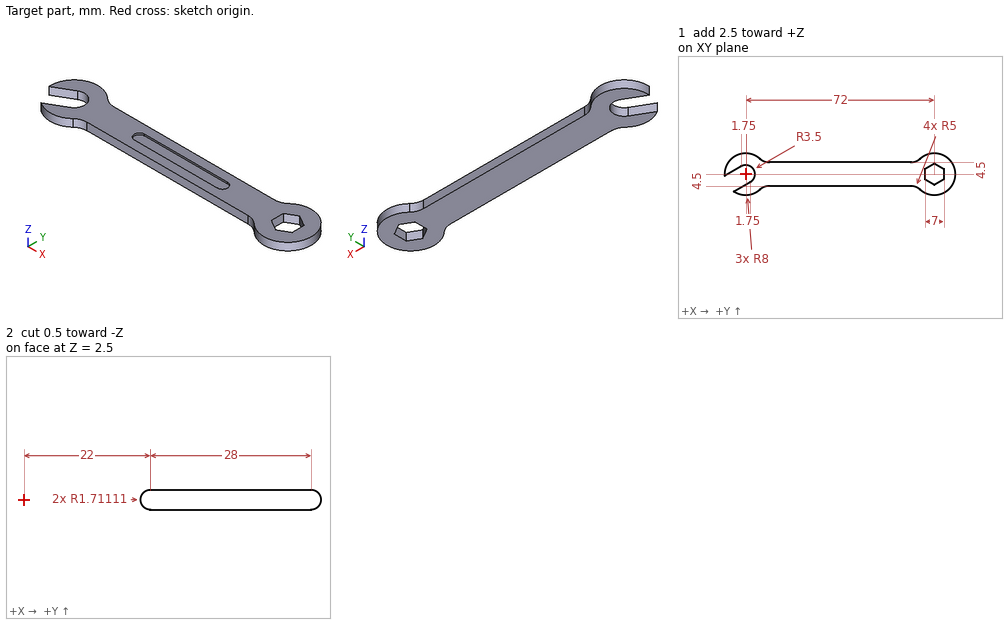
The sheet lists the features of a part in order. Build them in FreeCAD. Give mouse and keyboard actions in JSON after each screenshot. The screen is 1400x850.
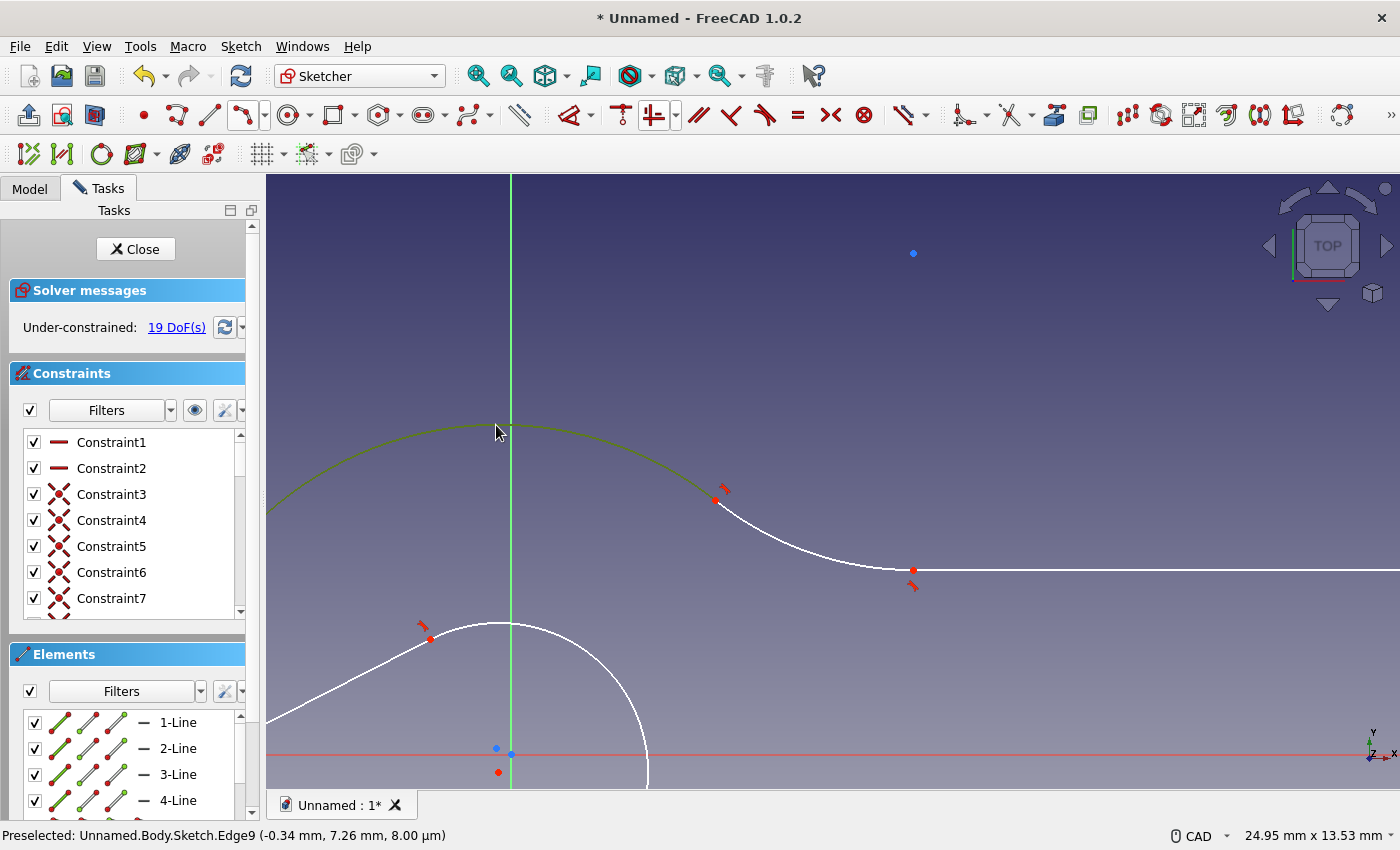
{"action": "scroll", "coordinate": [491, 424], "scroll_direction": "down", "scroll_amount": 9}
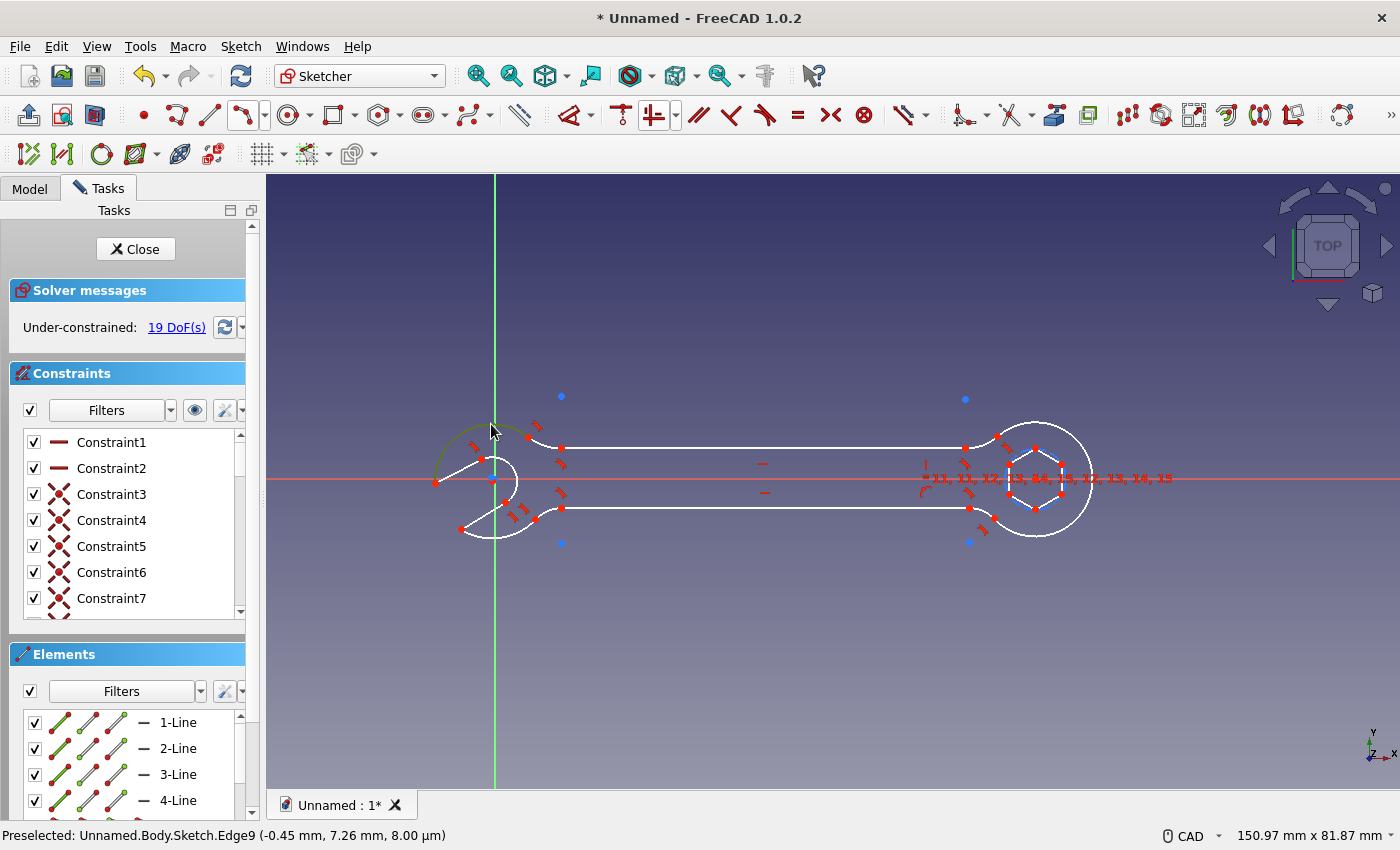
{"action": "scroll", "coordinate": [484, 538], "scroll_direction": "up", "scroll_amount": 2}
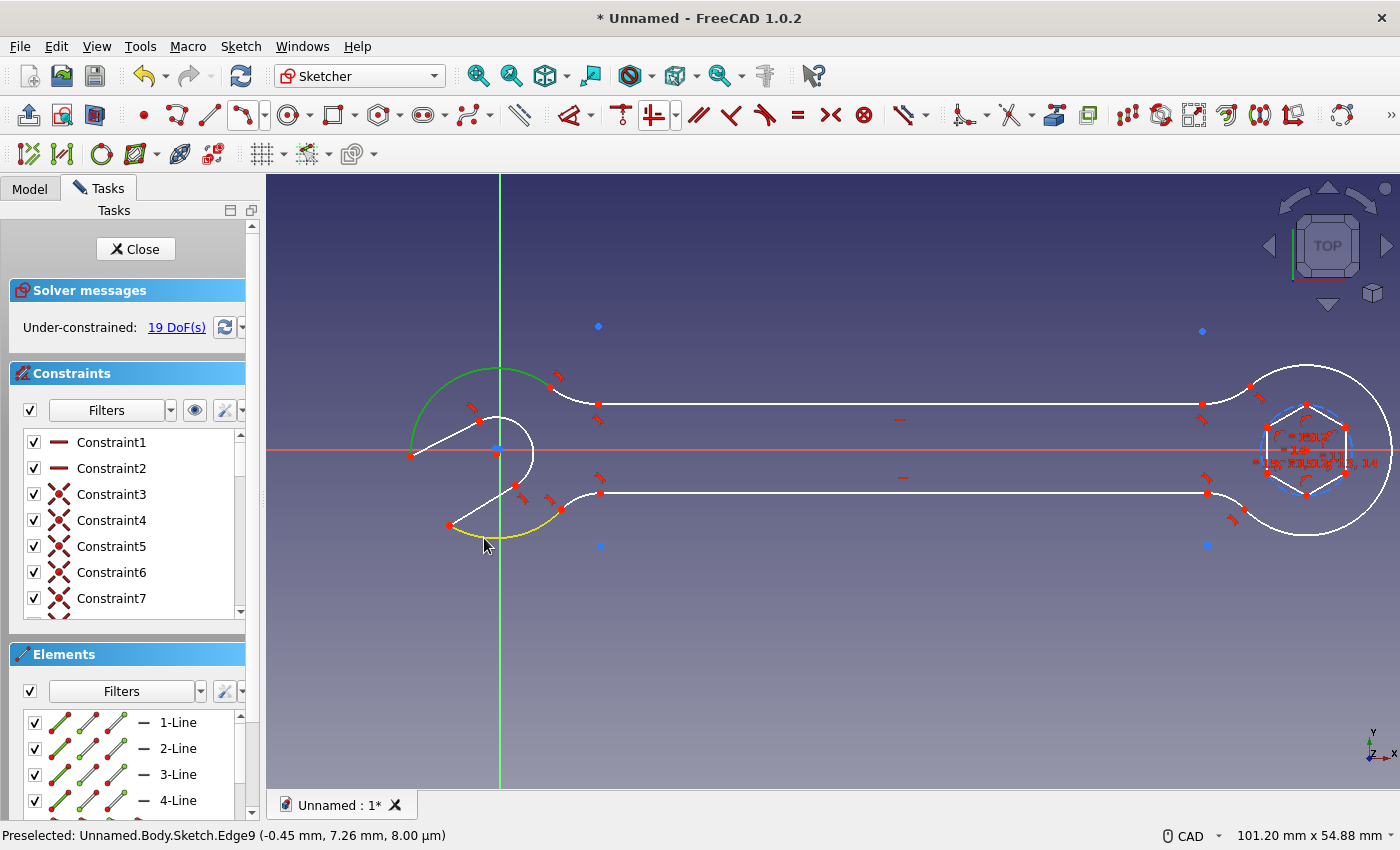
{"action": "left_click", "coordinate": [484, 537]}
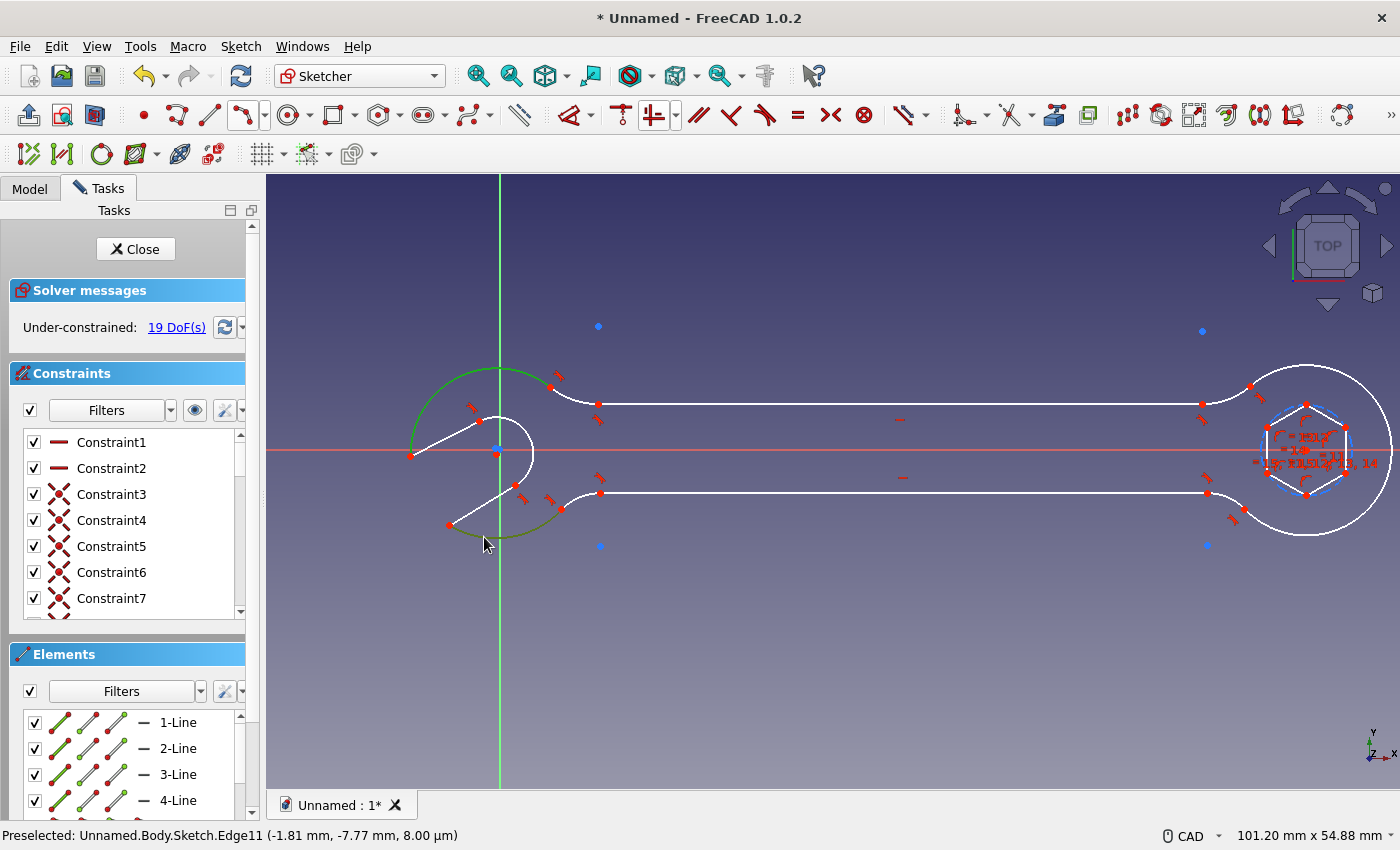
{"action": "left_click", "coordinate": [621, 116]}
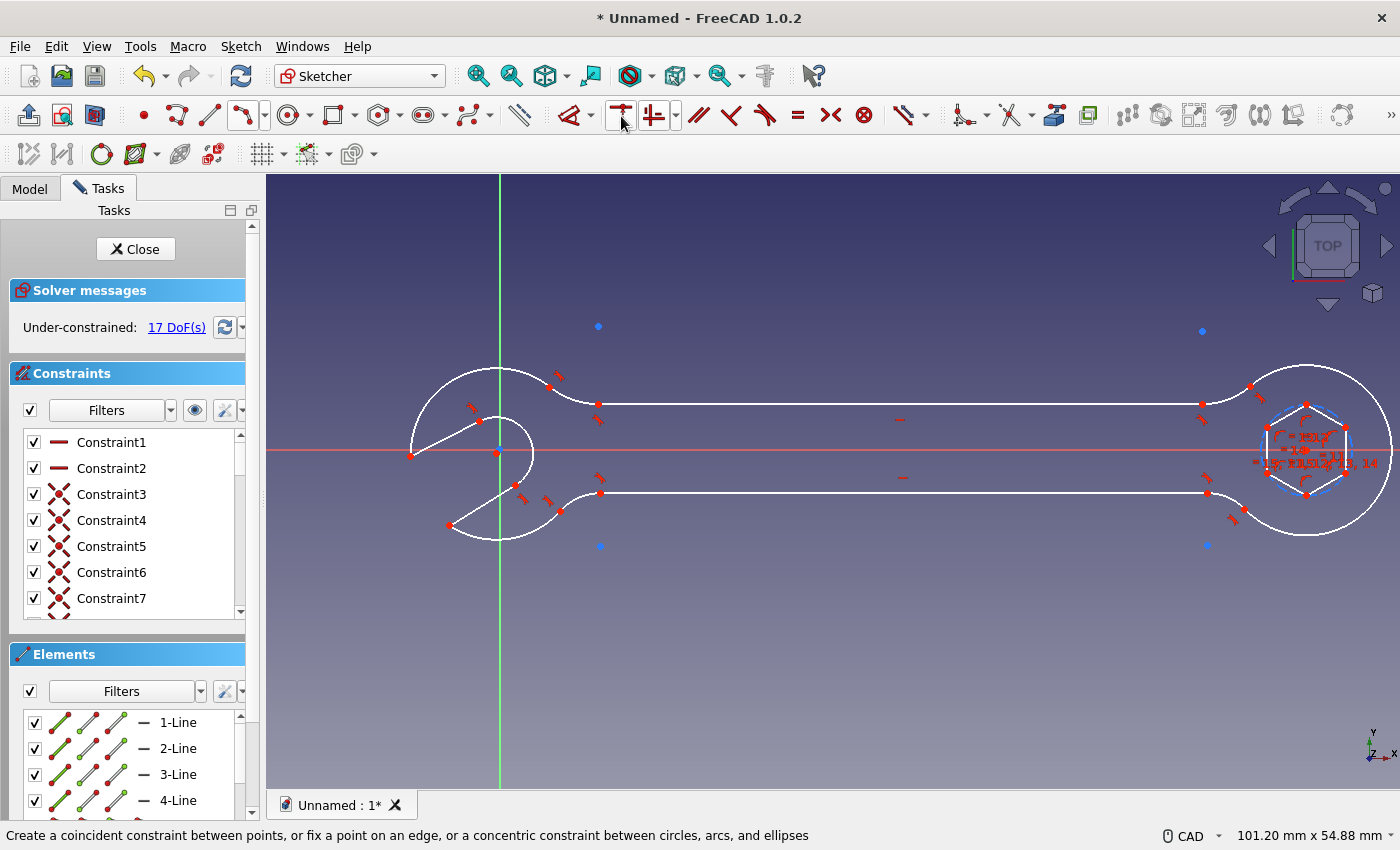
{"action": "left_click_drag", "start_coordinate": [486, 440], "coordinate": [510, 464]}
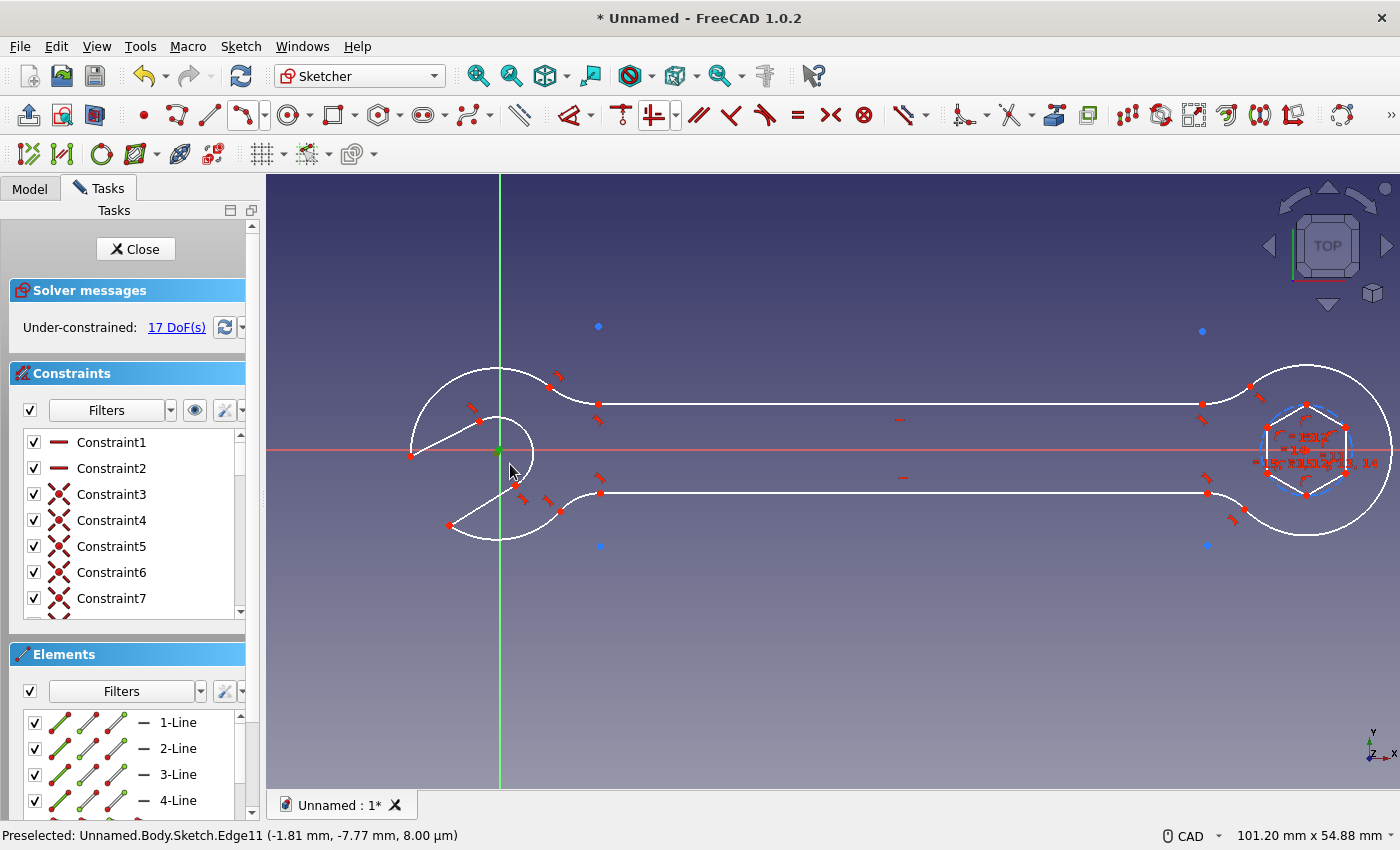
{"action": "left_click", "coordinate": [621, 116]}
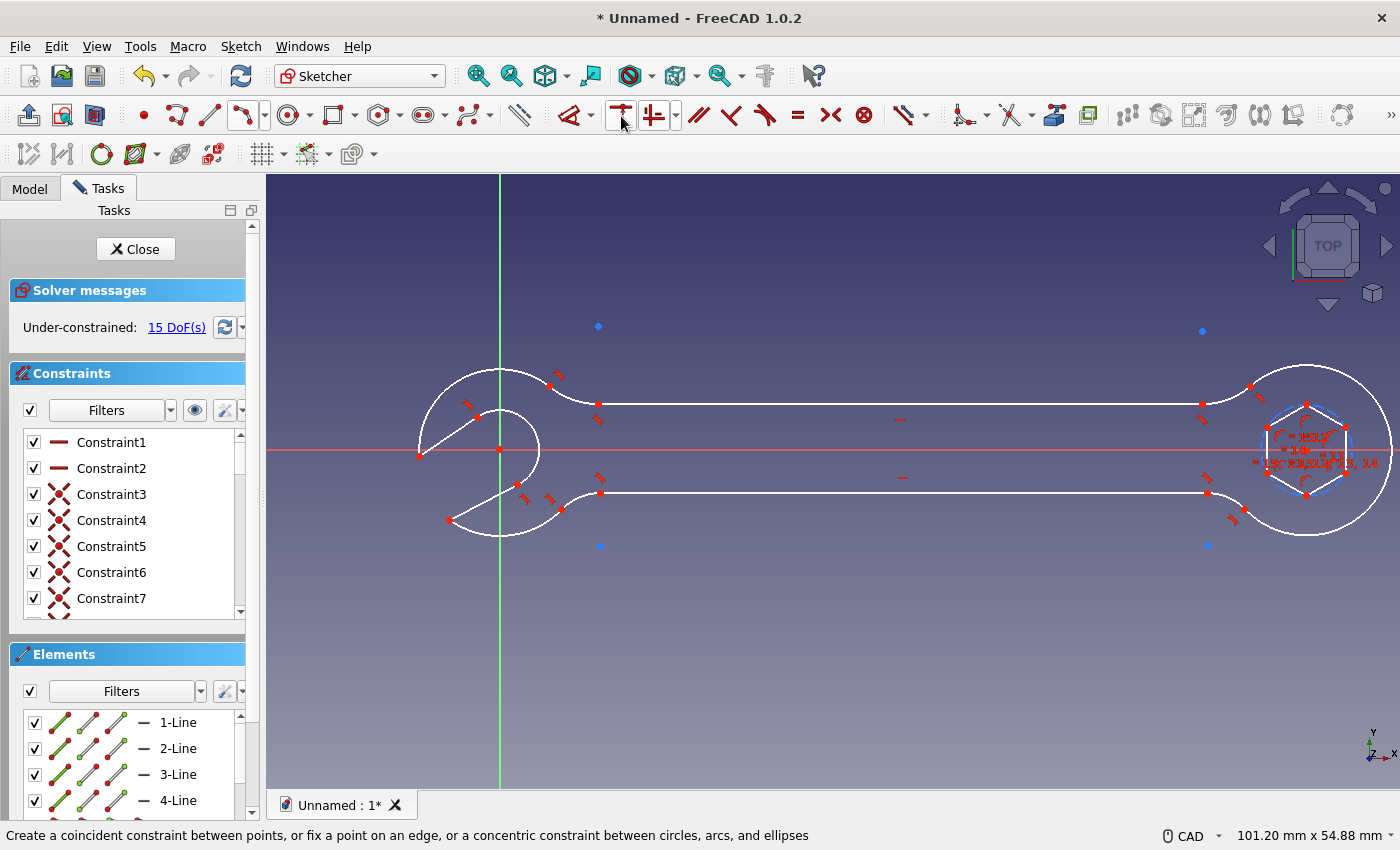
{"action": "left_click", "coordinate": [1220, 495]}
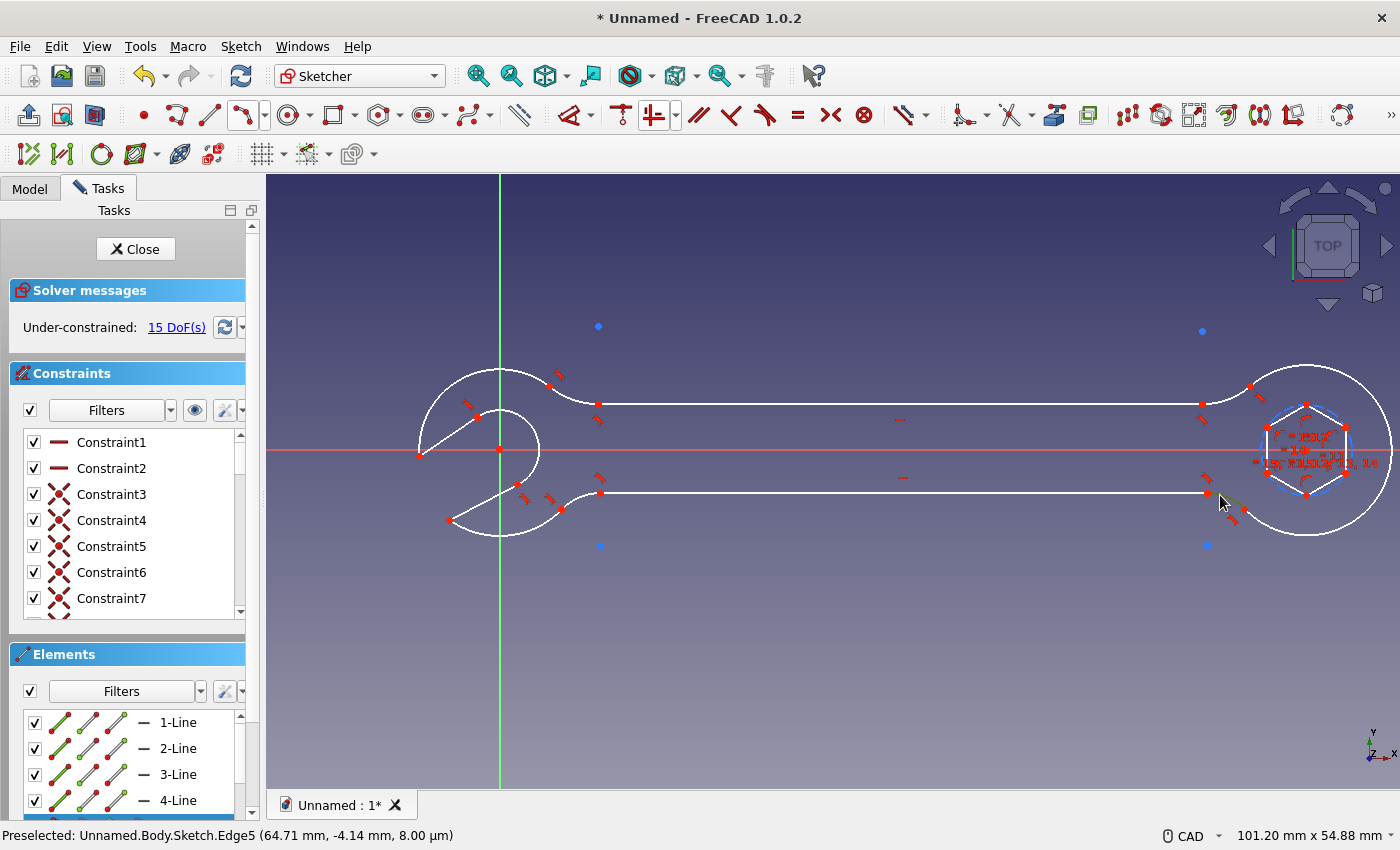
{"action": "left_click", "coordinate": [1218, 402]}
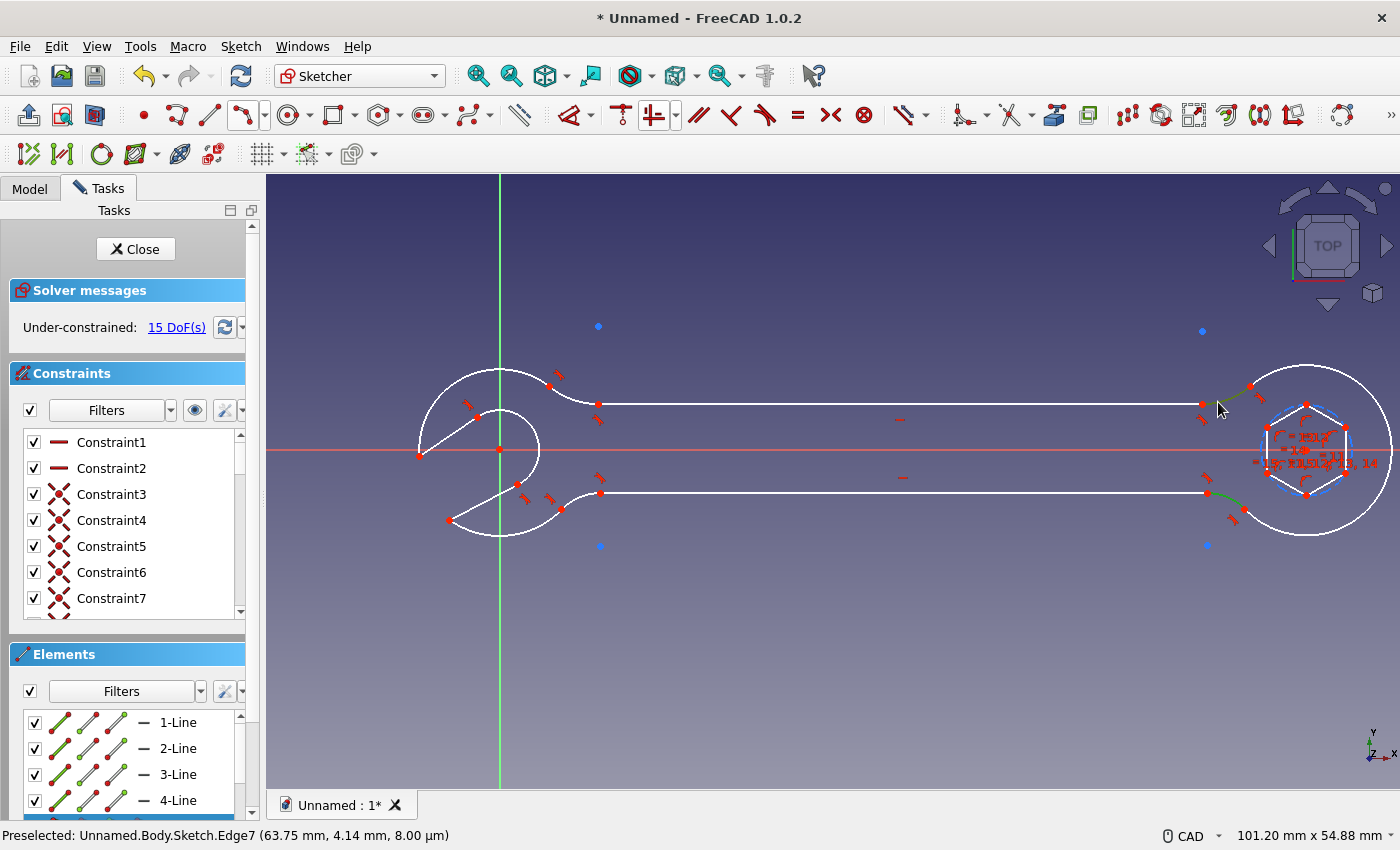
{"action": "left_click", "coordinate": [563, 396]}